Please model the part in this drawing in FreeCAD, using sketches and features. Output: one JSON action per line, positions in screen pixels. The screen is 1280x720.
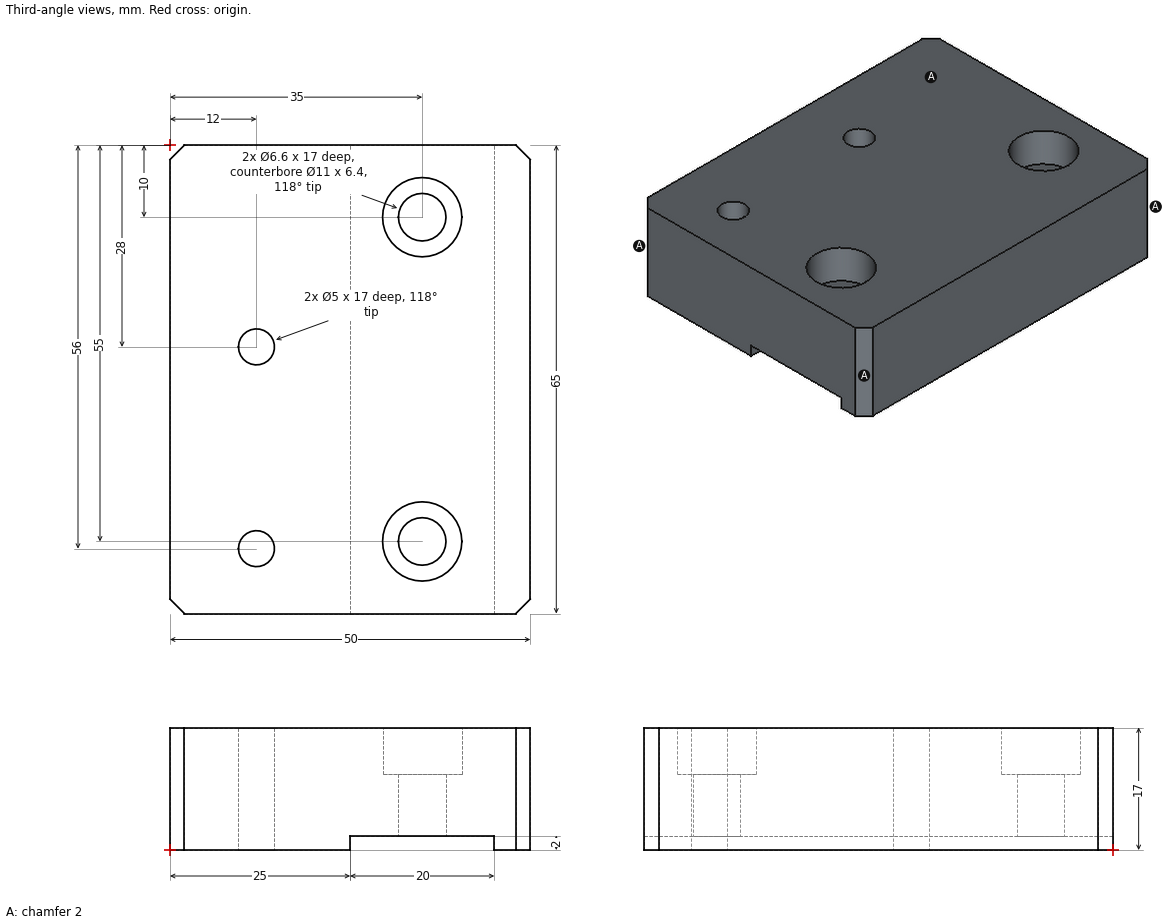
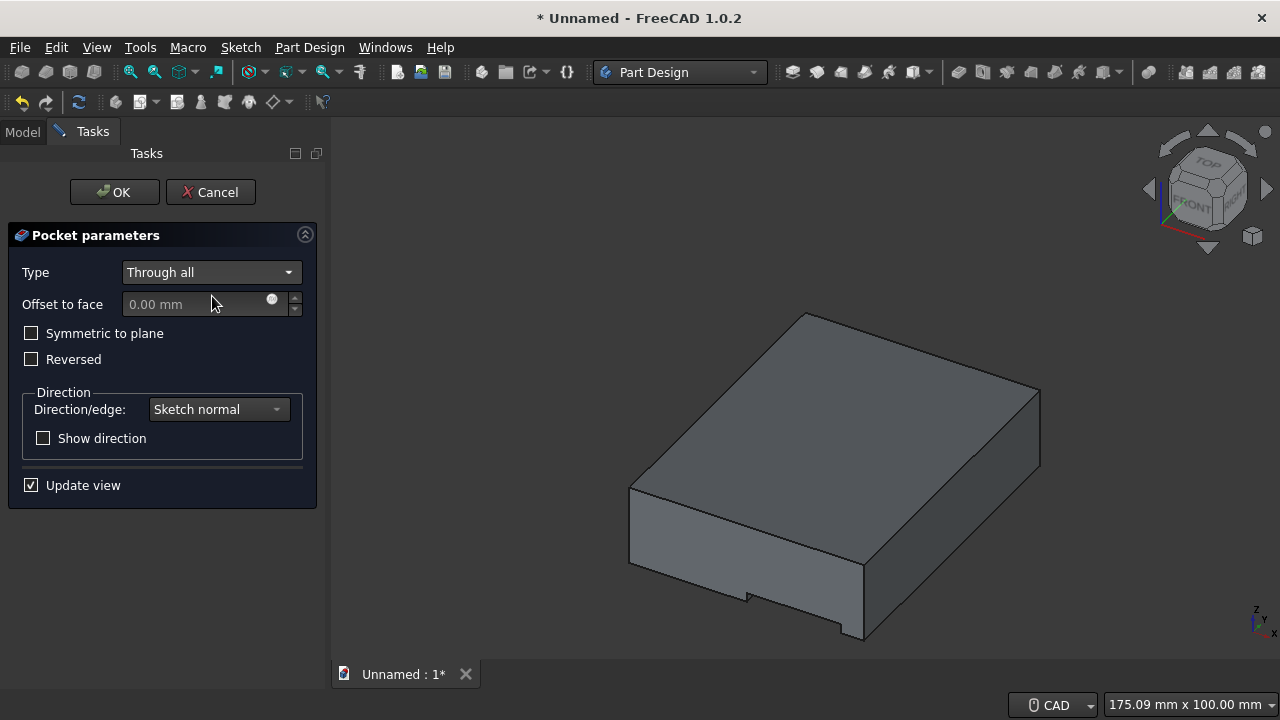
{"action": "left_click", "coordinate": [115, 192]}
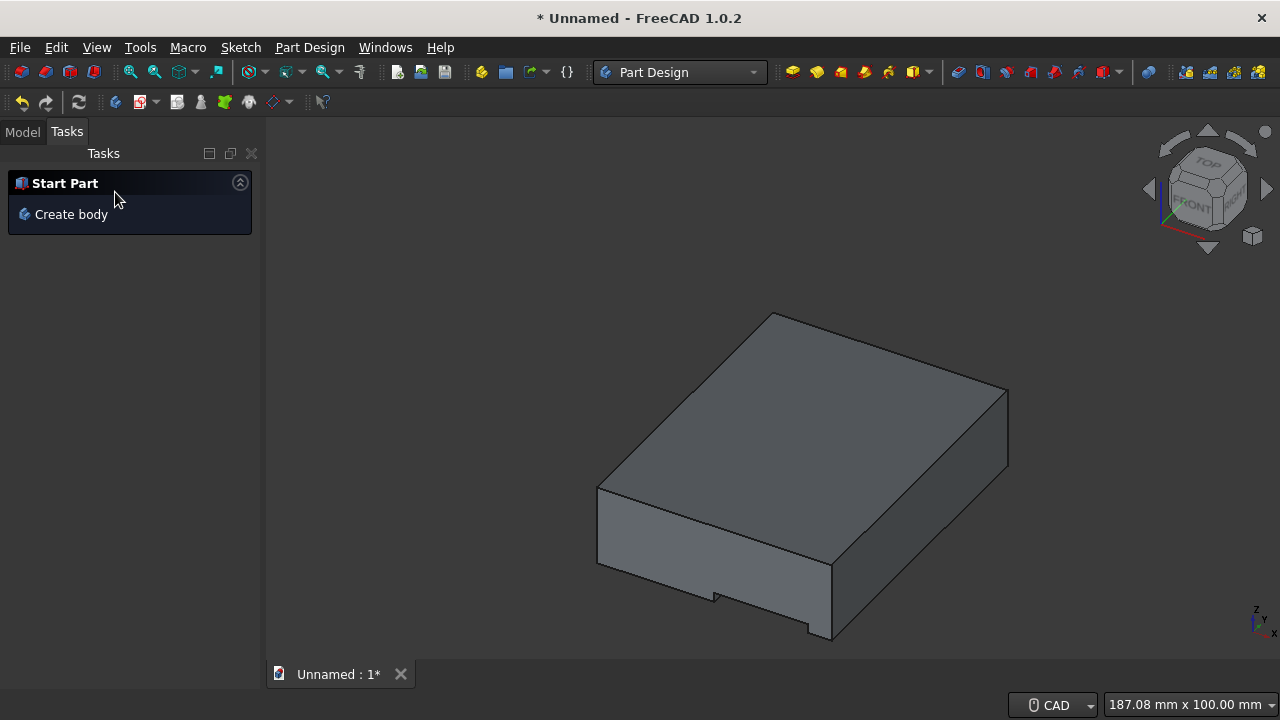
{"action": "left_click", "coordinate": [832, 602]}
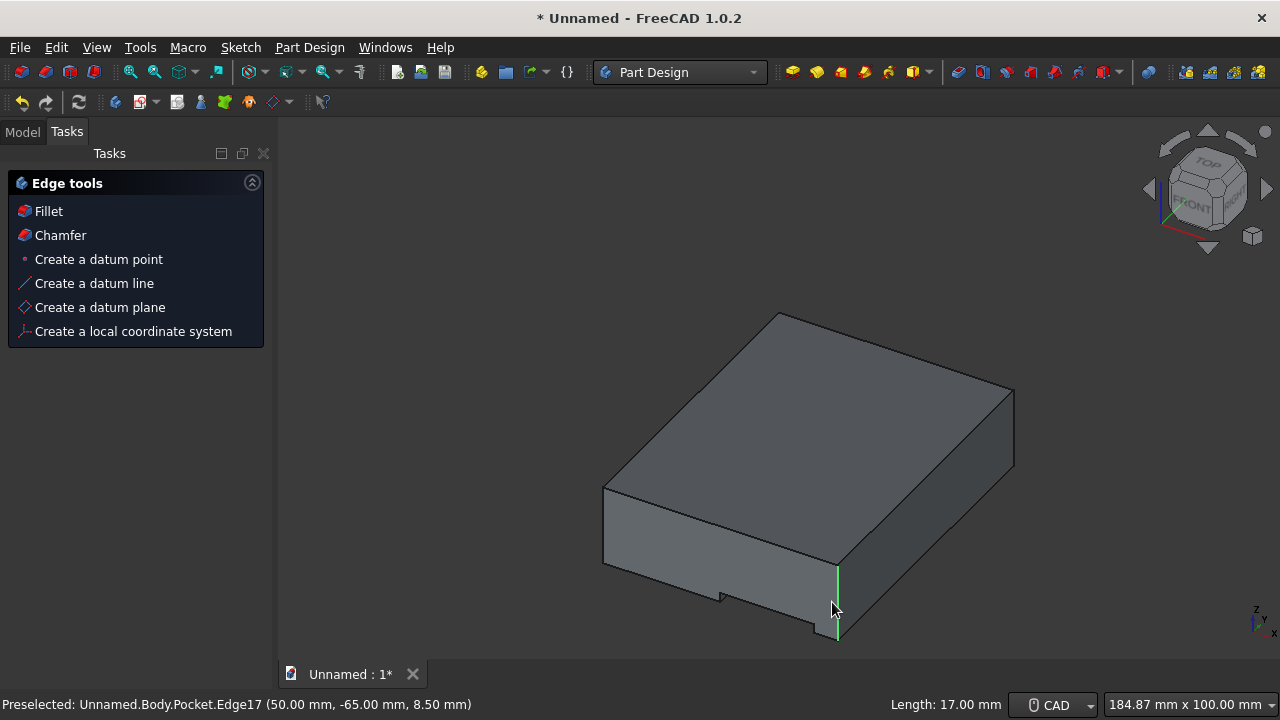
{"action": "key", "text": "0"}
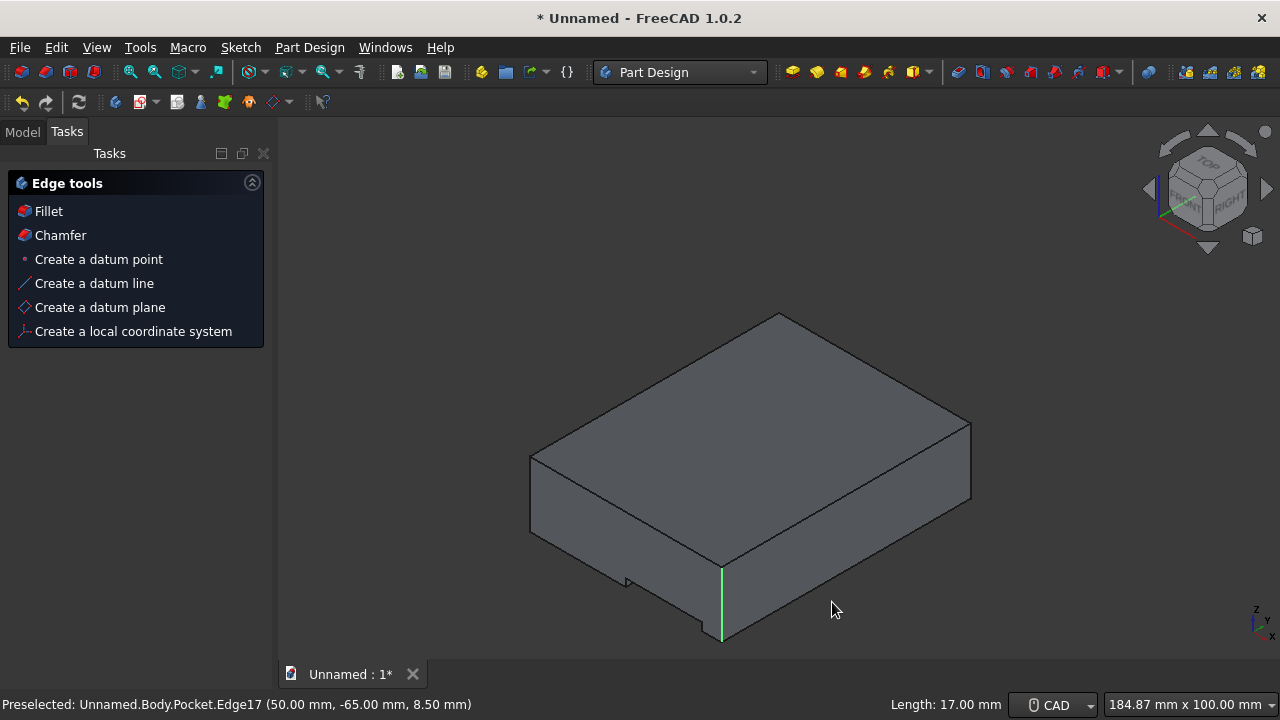
{"action": "key", "text": "2"}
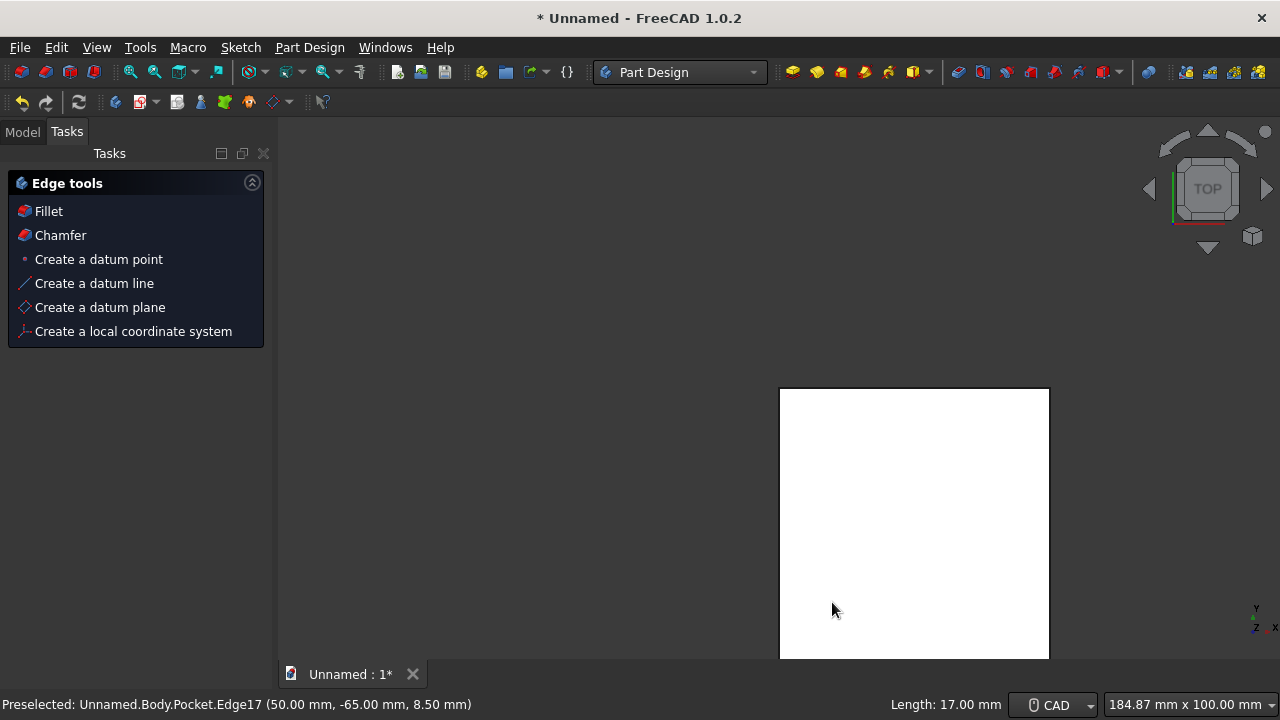
{"action": "left_click", "coordinate": [132, 72]}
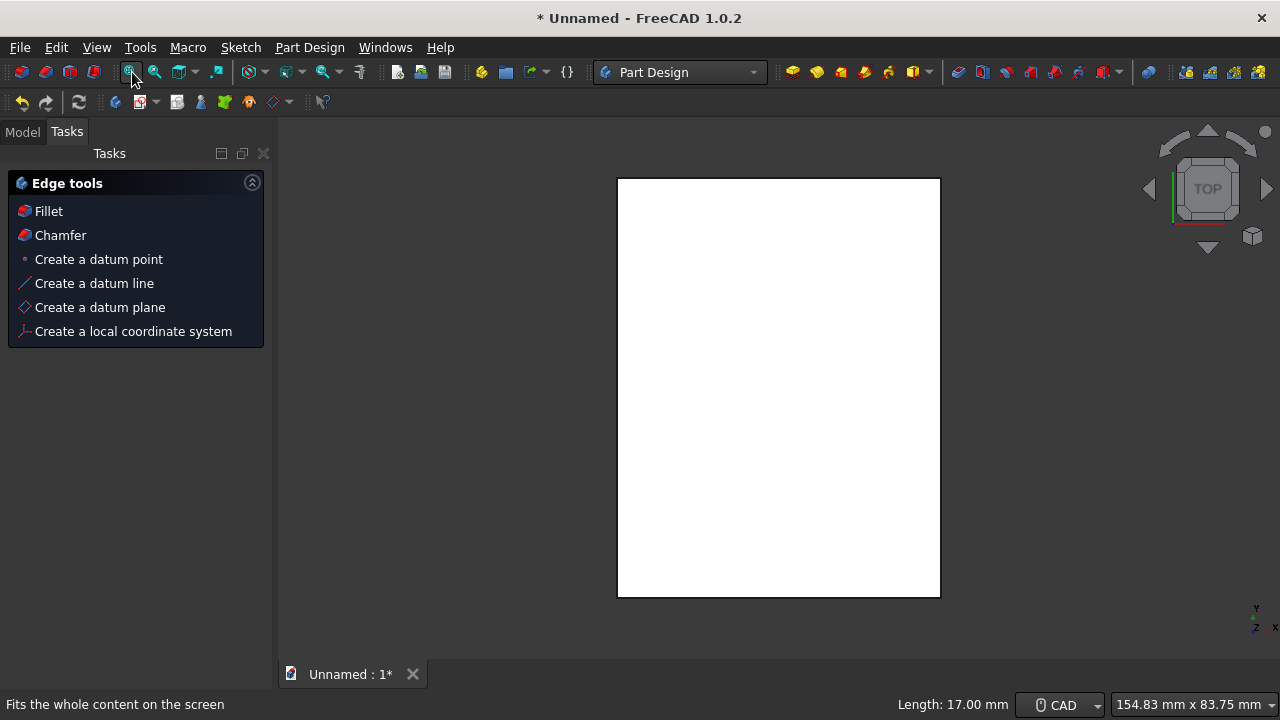
{"action": "key", "text": "1"}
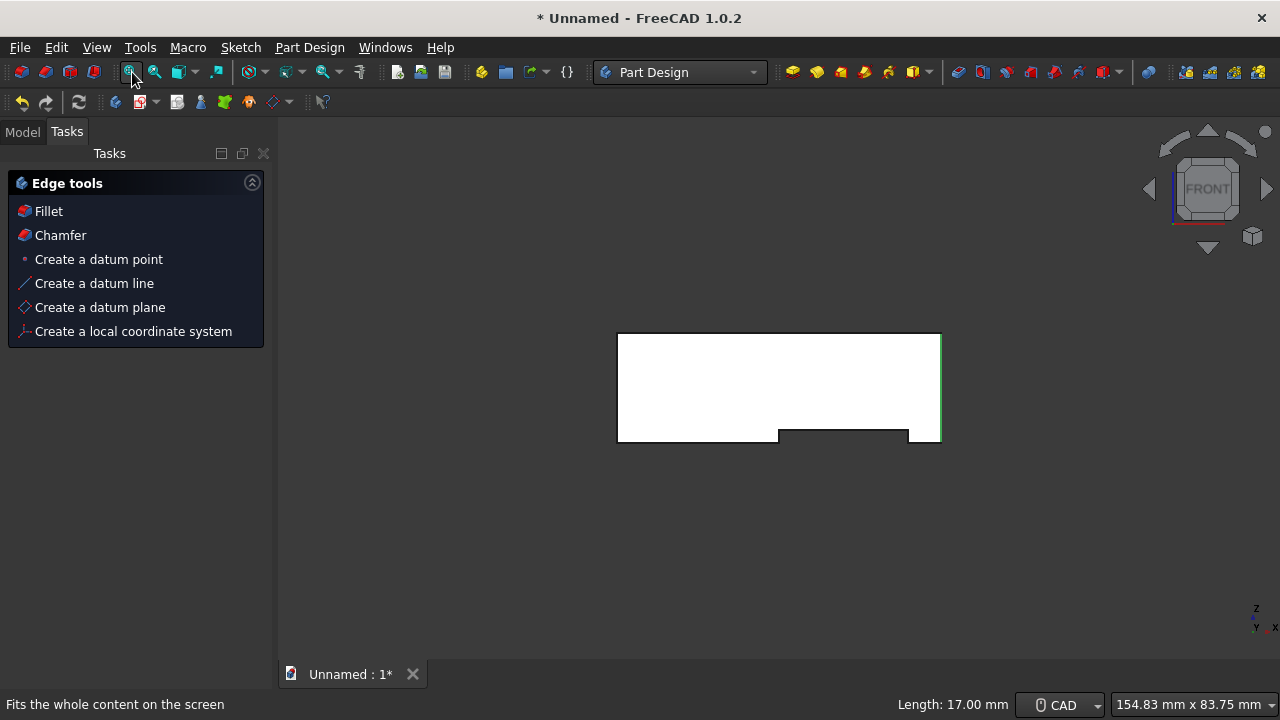
{"action": "left_click", "coordinate": [132, 72]}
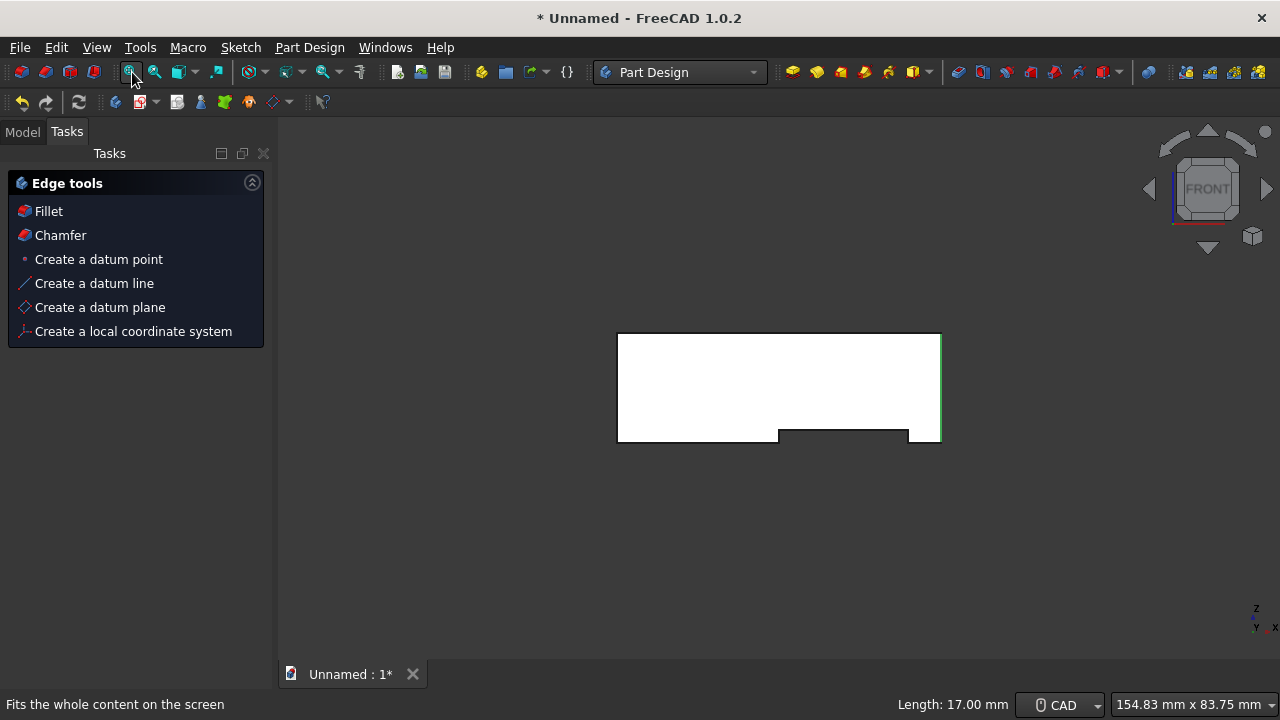
{"action": "left_click", "coordinate": [617, 387], "text": "ctrl"}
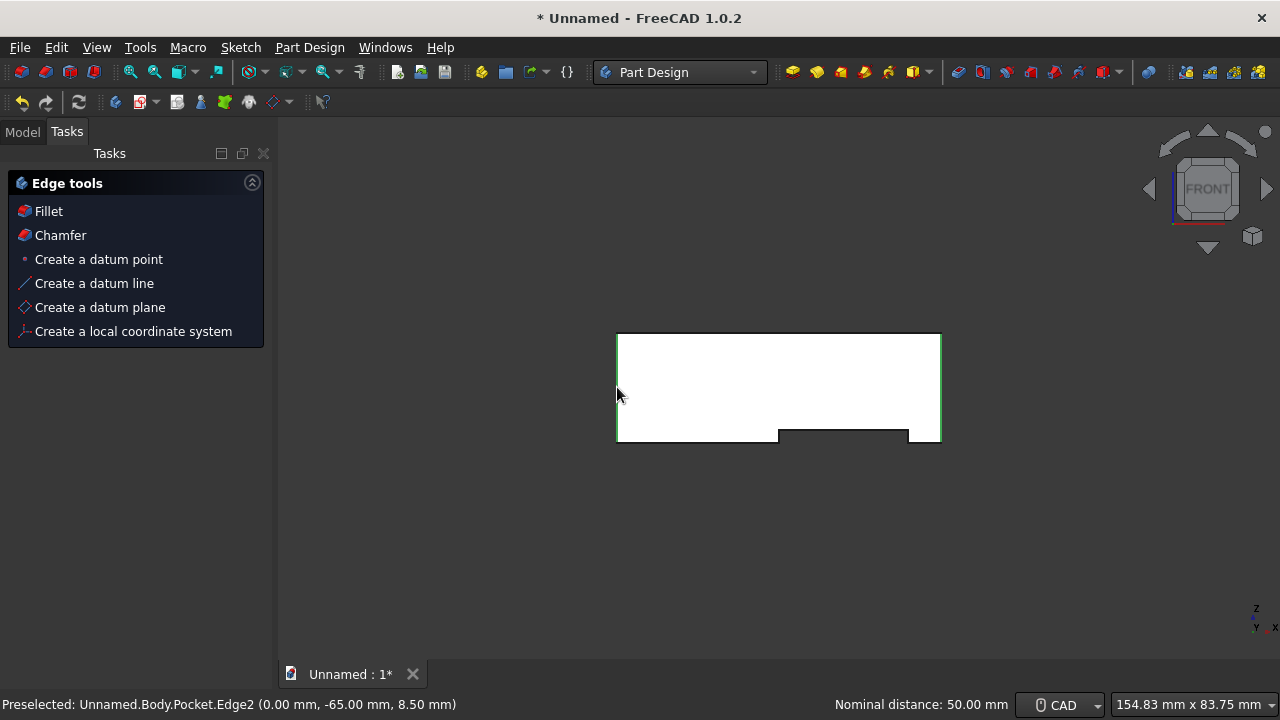
{"action": "key", "text": "3"}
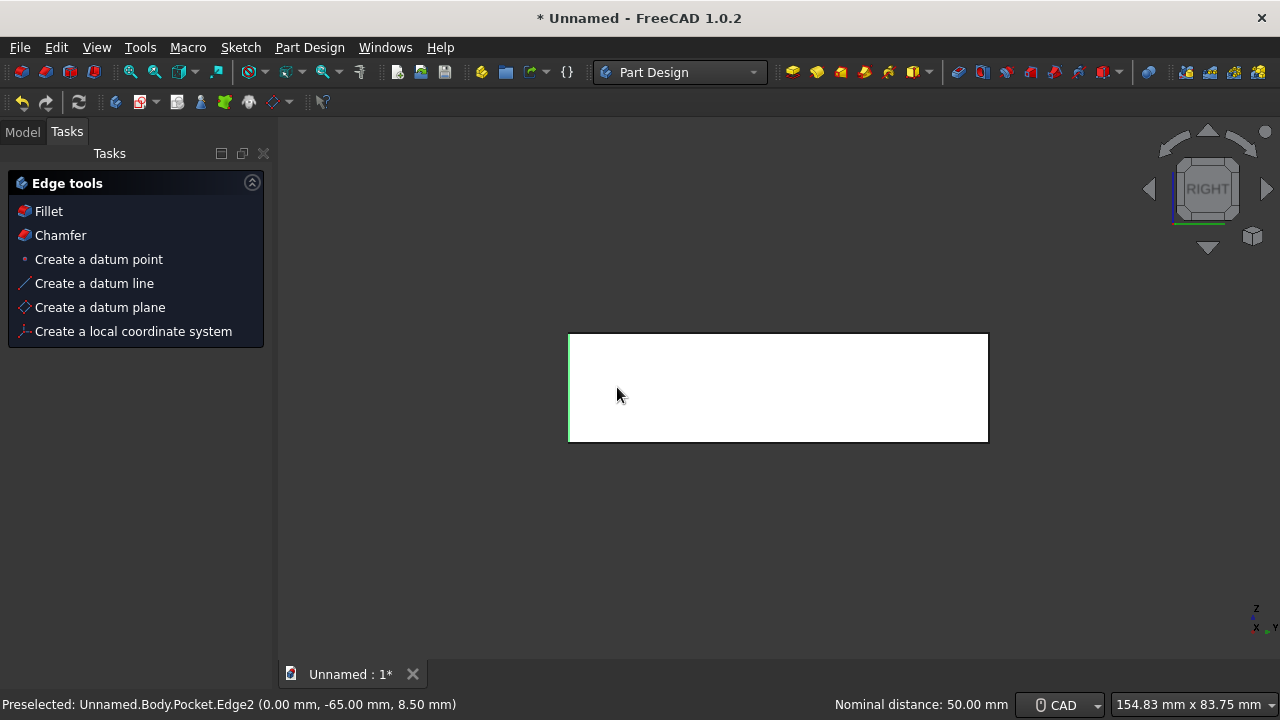
{"action": "left_click", "coordinate": [132, 72]}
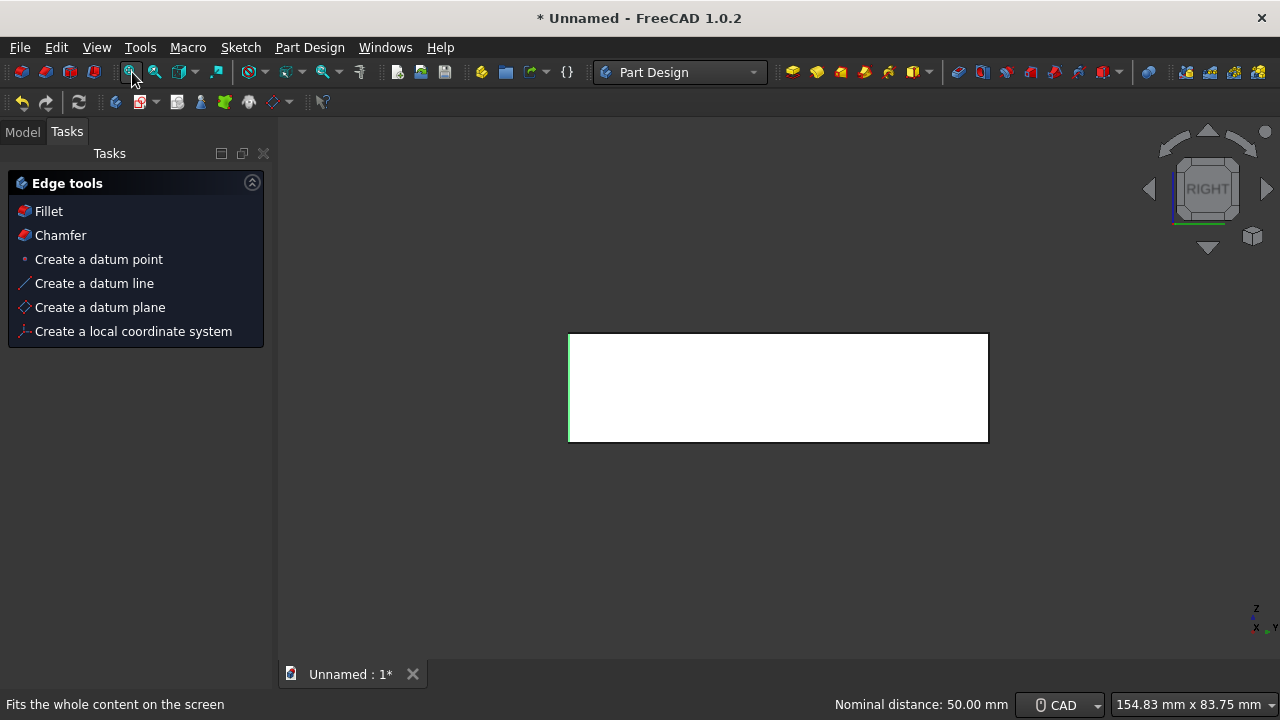
{"action": "left_click", "coordinate": [989, 387], "text": "ctrl"}